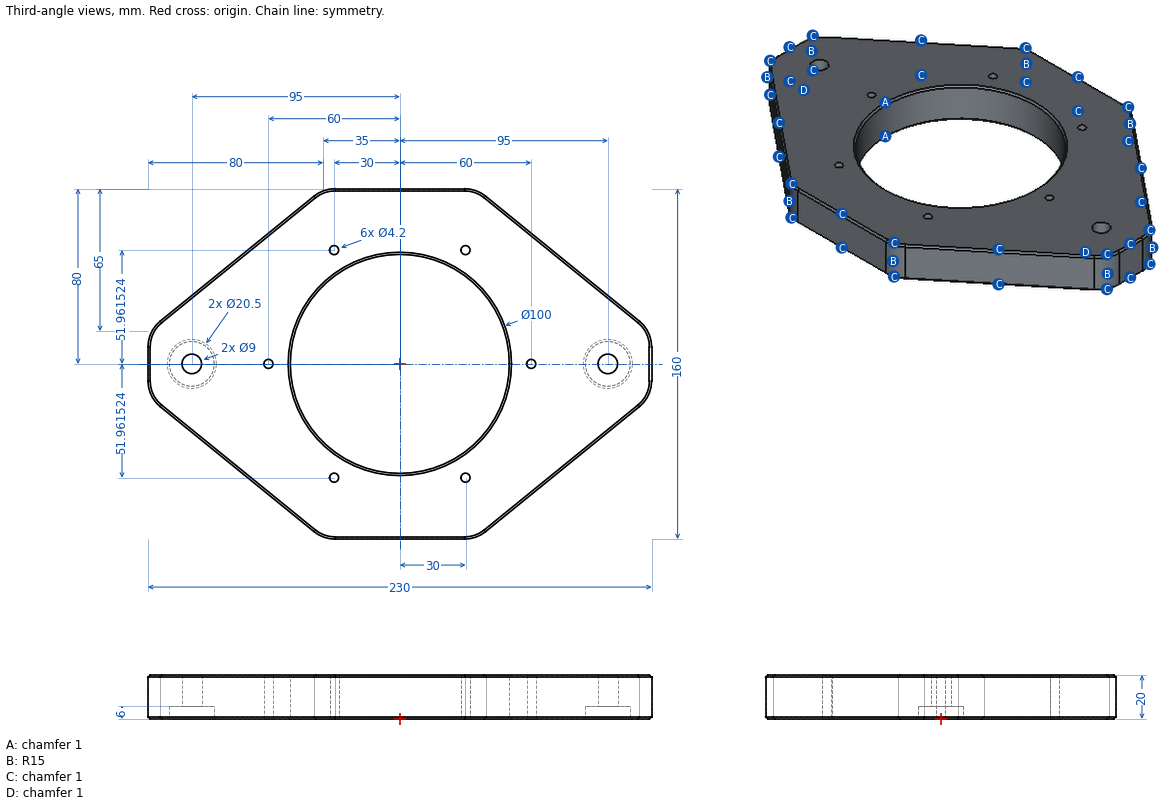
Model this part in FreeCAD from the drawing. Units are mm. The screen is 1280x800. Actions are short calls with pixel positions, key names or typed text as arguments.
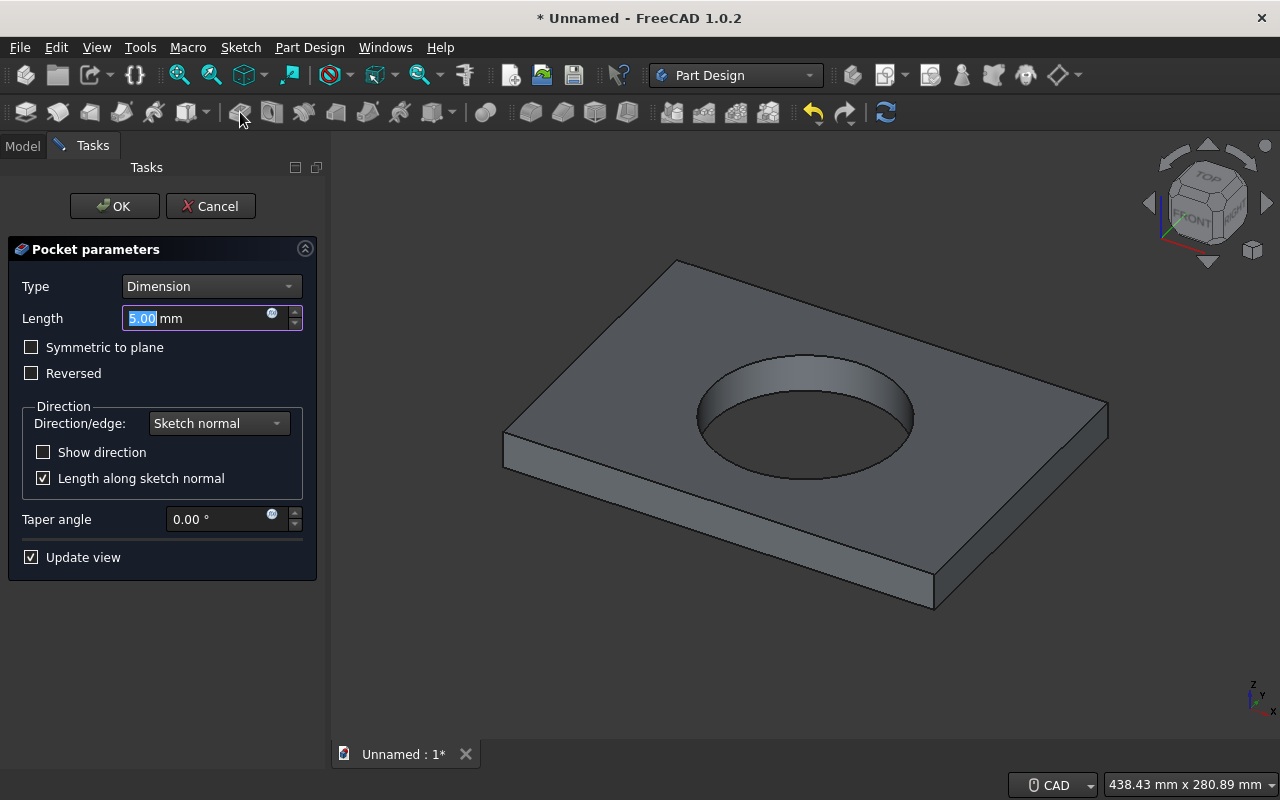
text(6)
key(Tab)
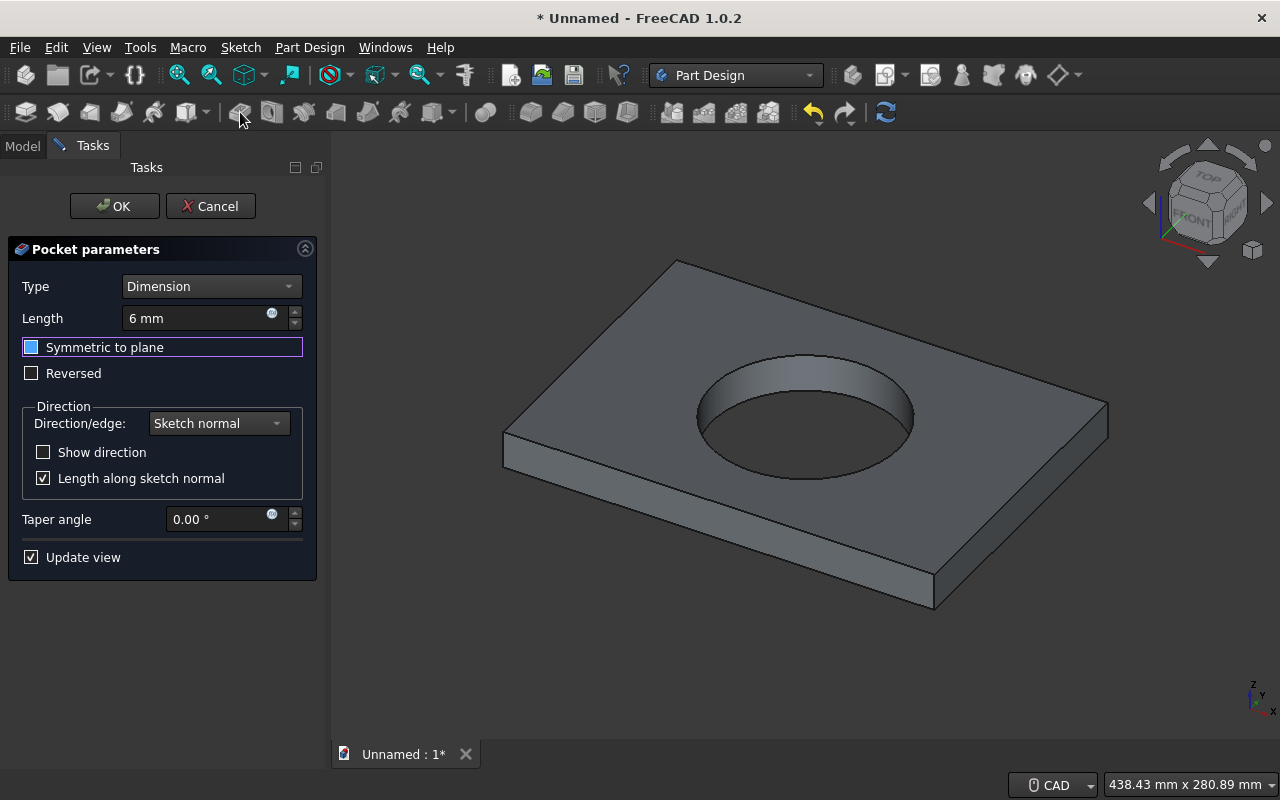
click(30, 373)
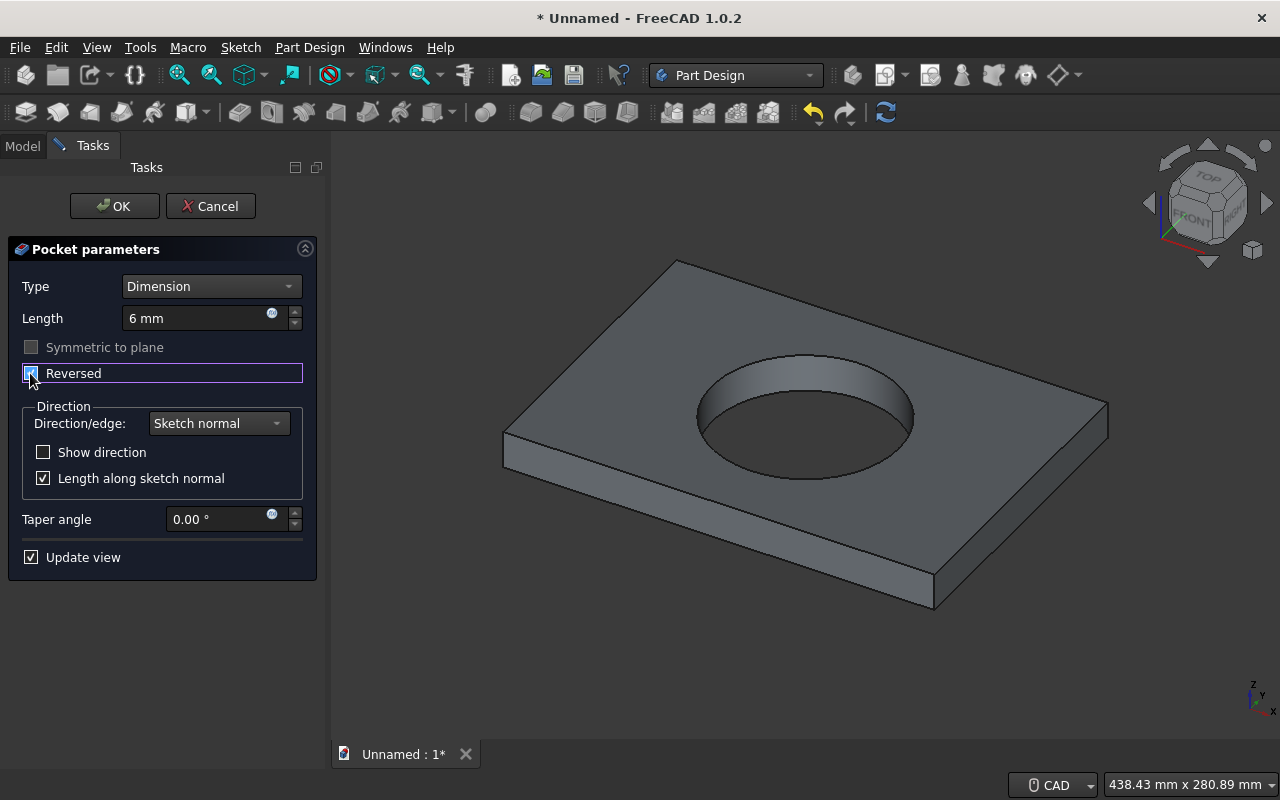
click(115, 206)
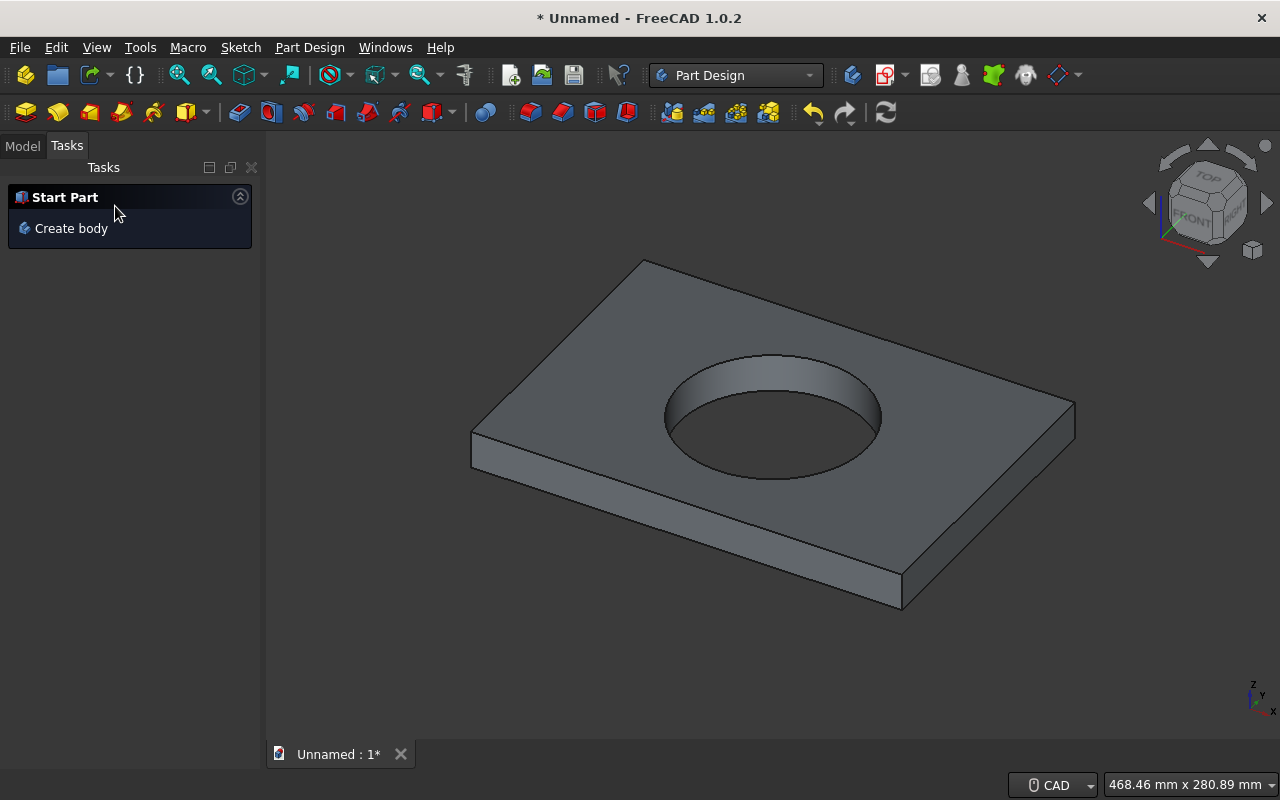
click(946, 408)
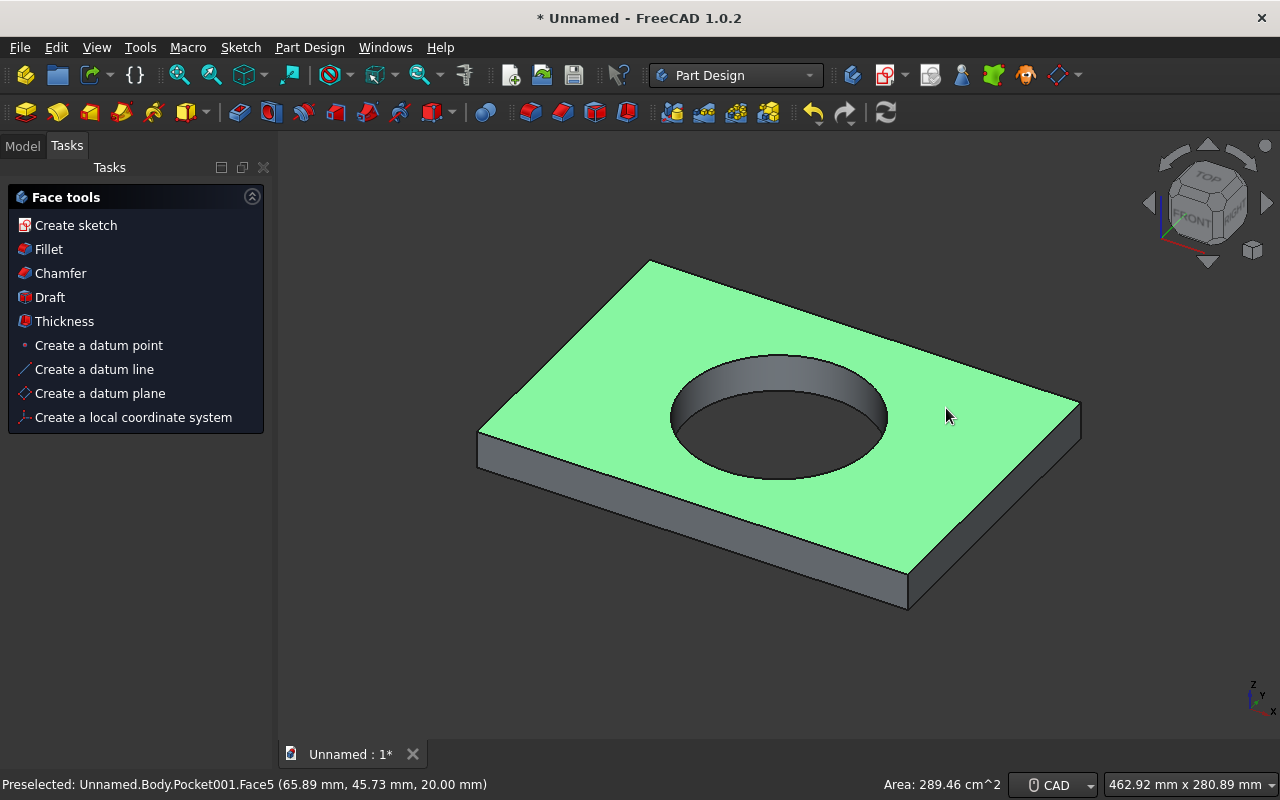
click(886, 76)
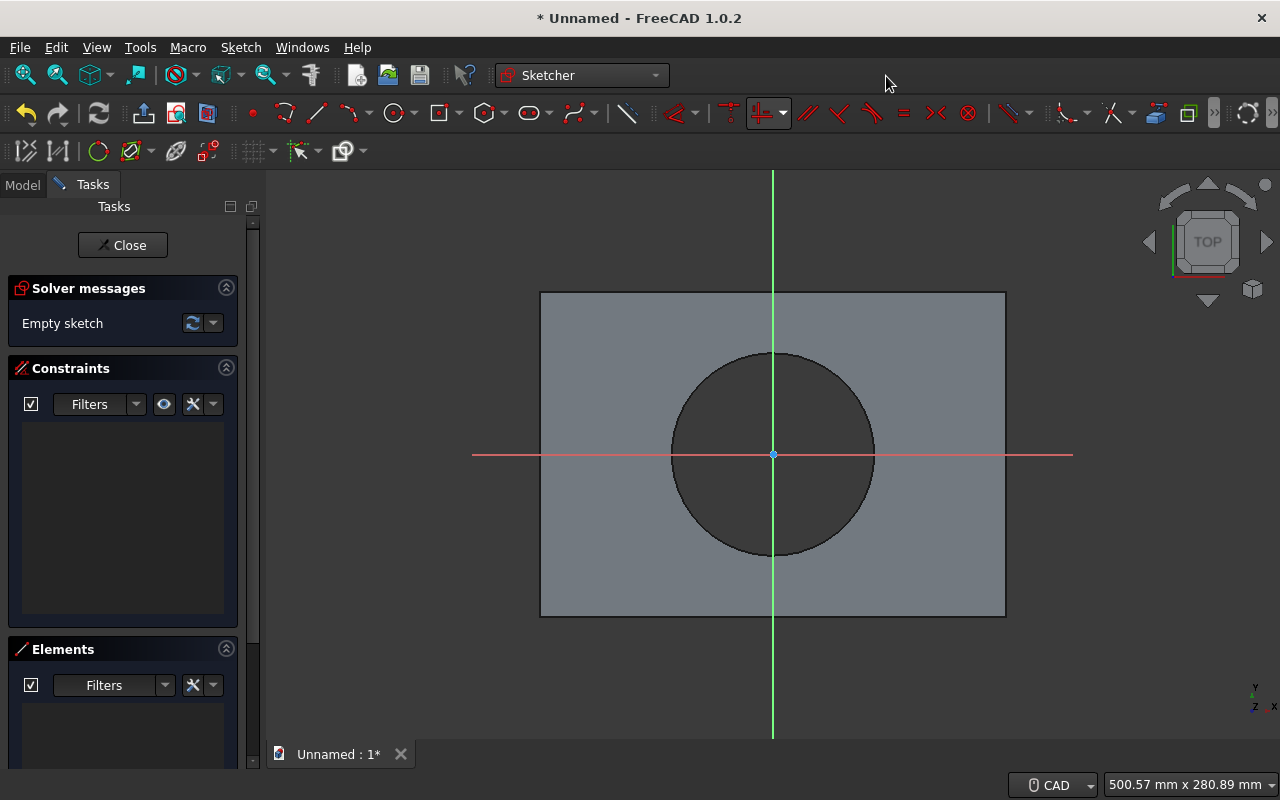
scroll(912, 455, up, 2)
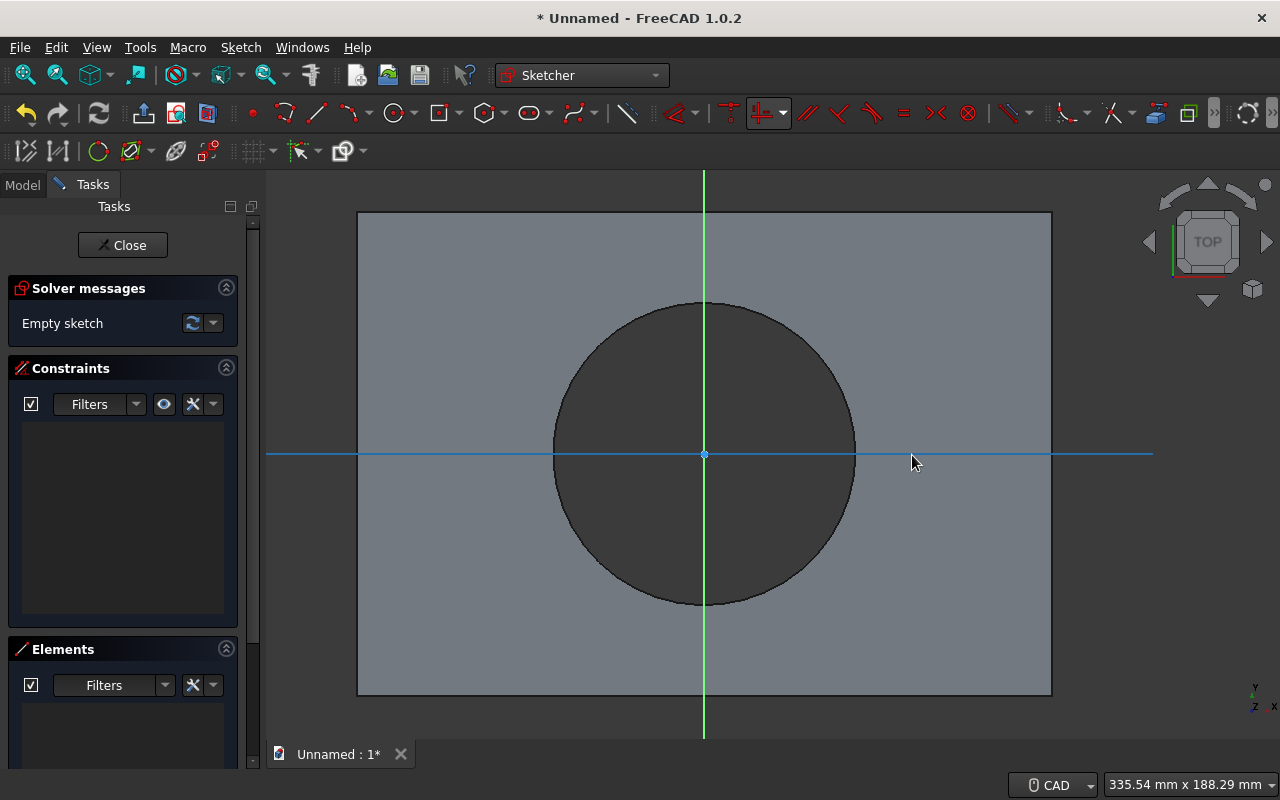
click(394, 114)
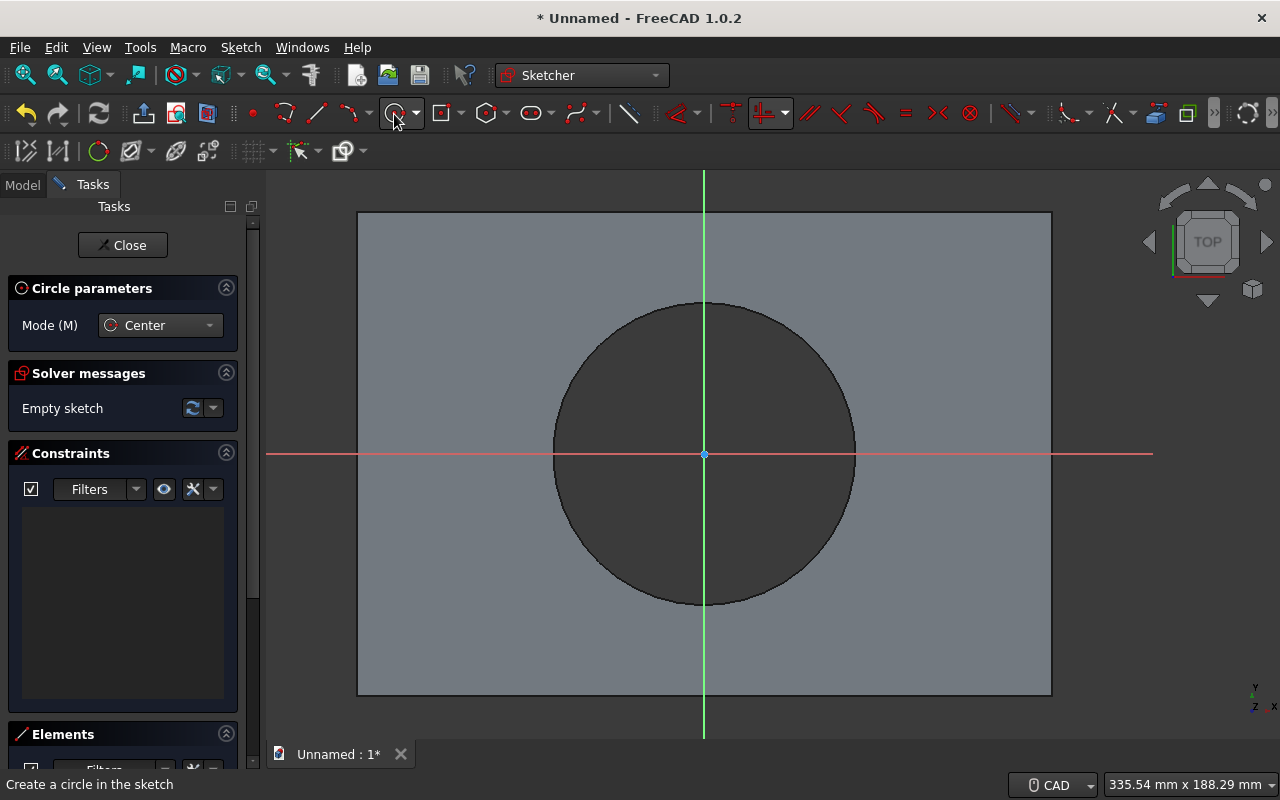
scroll(417, 454, up, 3)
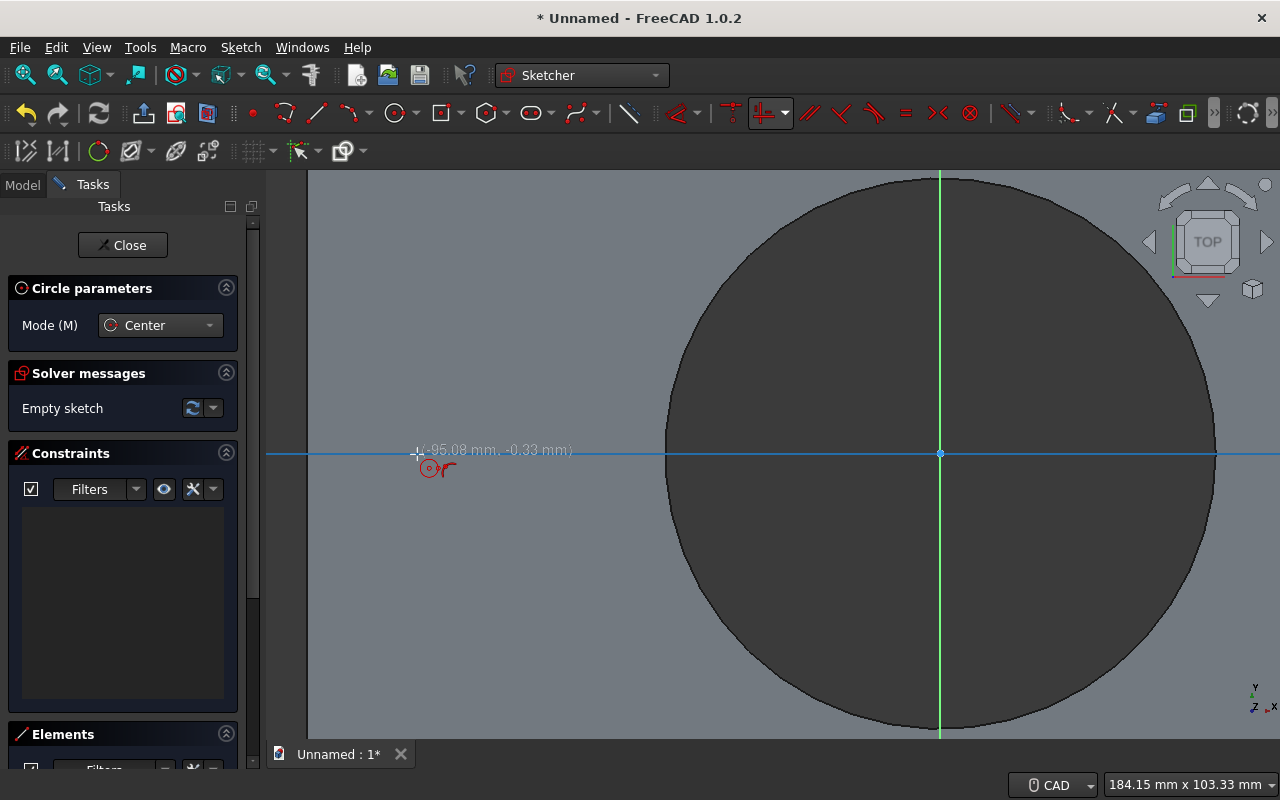
click(417, 454)
move(435, 436)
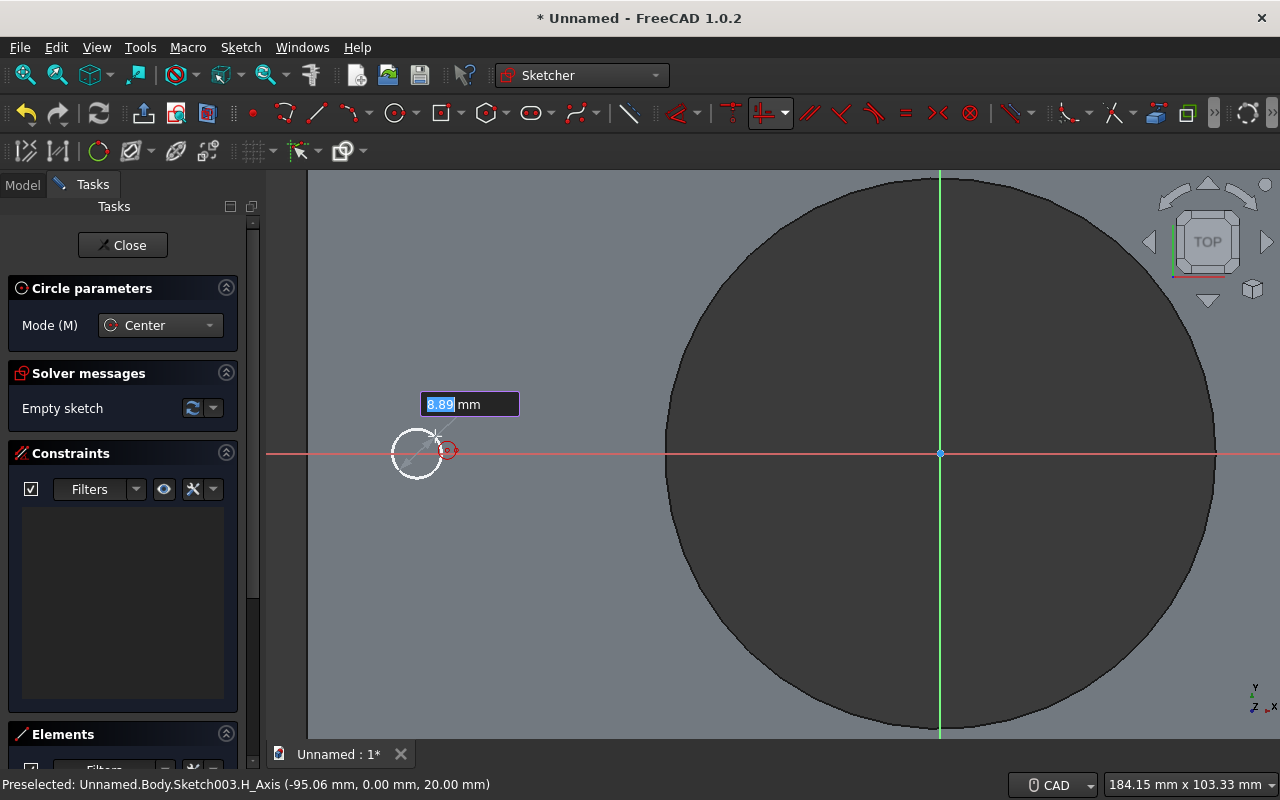
text(9)
key(Return)